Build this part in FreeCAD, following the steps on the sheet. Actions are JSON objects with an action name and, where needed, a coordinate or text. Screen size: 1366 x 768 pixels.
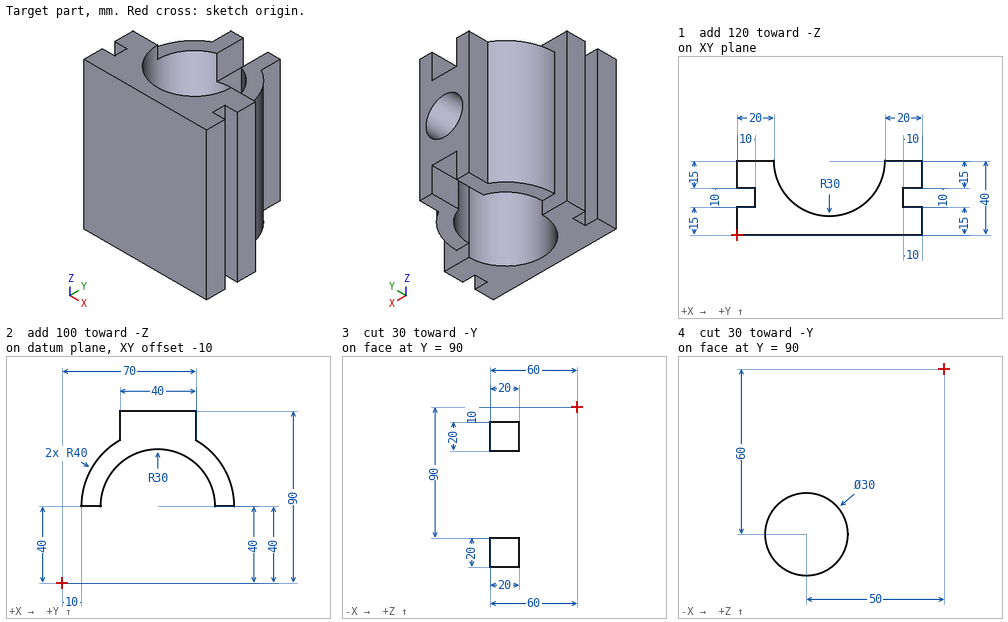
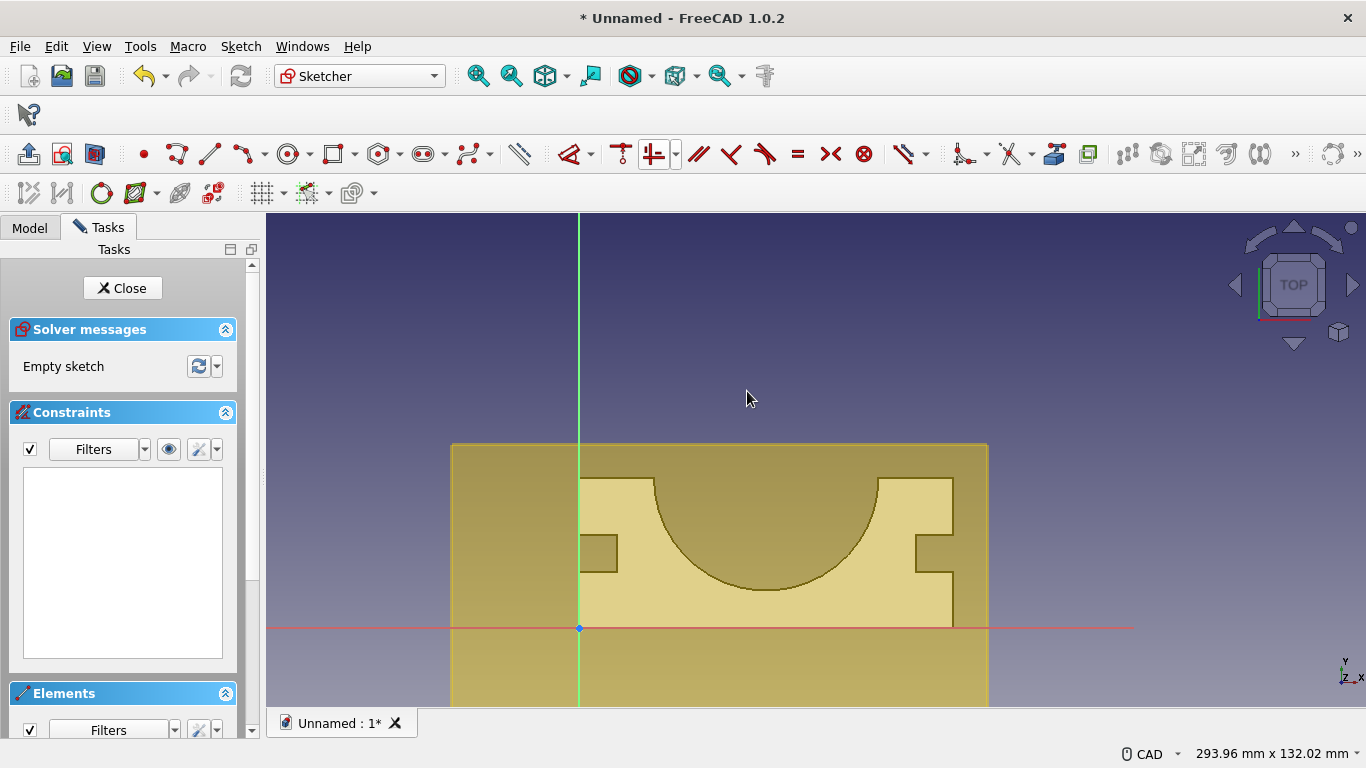
{"action": "left_click", "coordinate": [210, 154]}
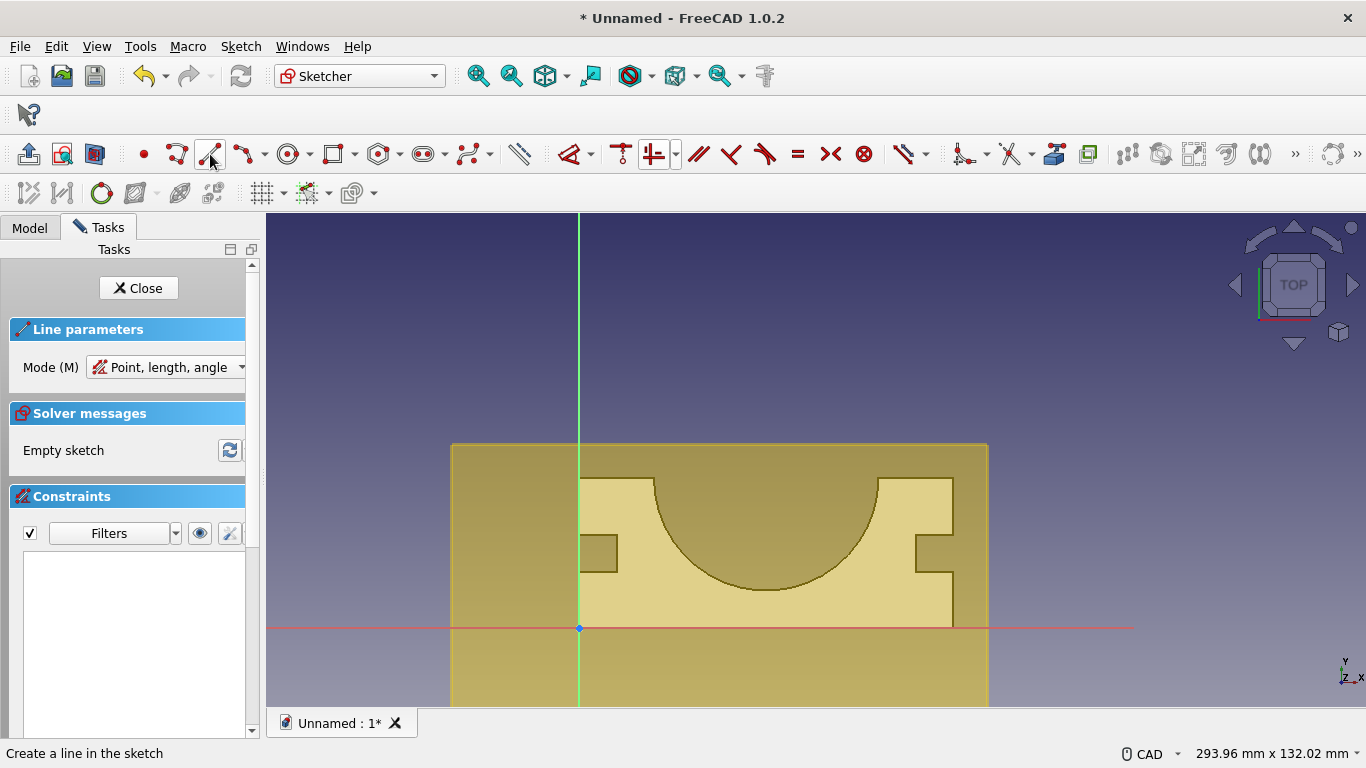
{"action": "left_click", "coordinate": [617, 478]}
{"action": "left_click", "coordinate": [654, 478]}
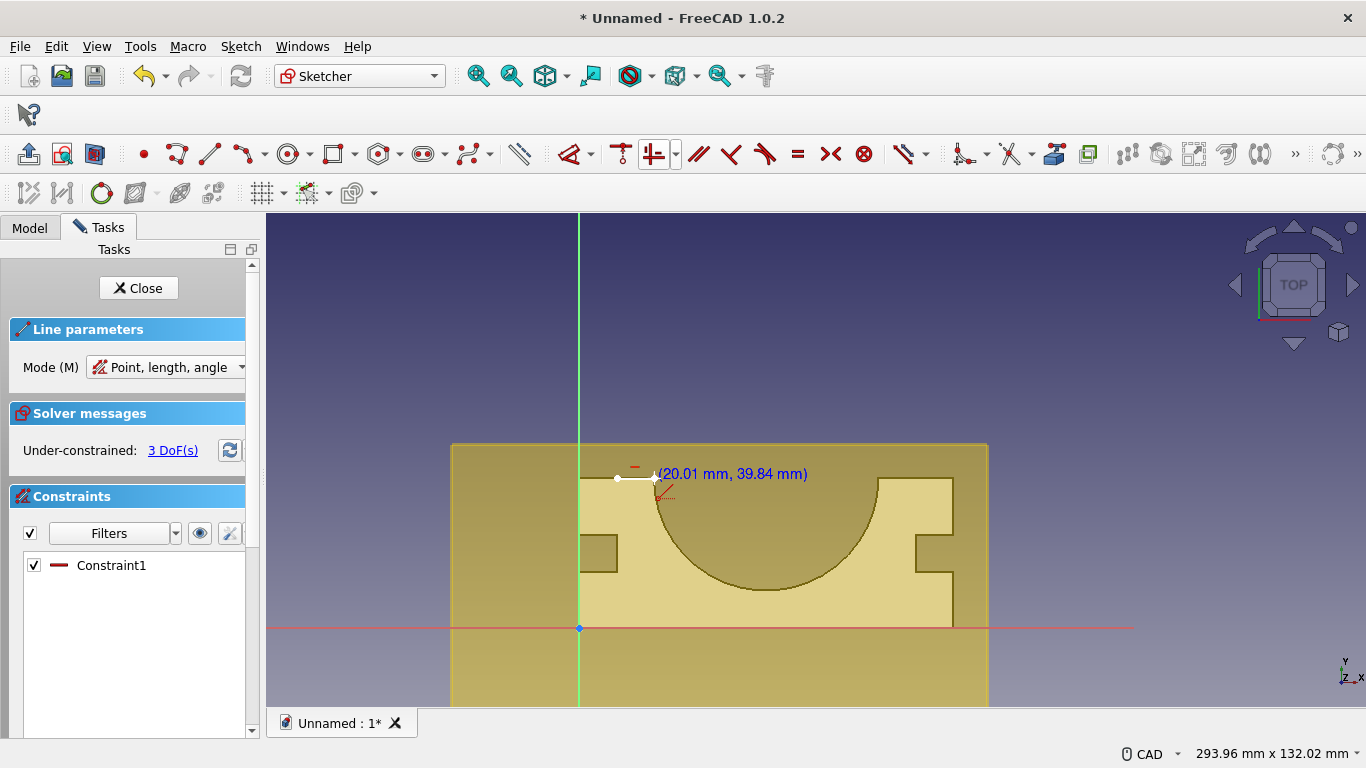
{"action": "left_click", "coordinate": [878, 478]}
{"action": "left_click", "coordinate": [916, 478]}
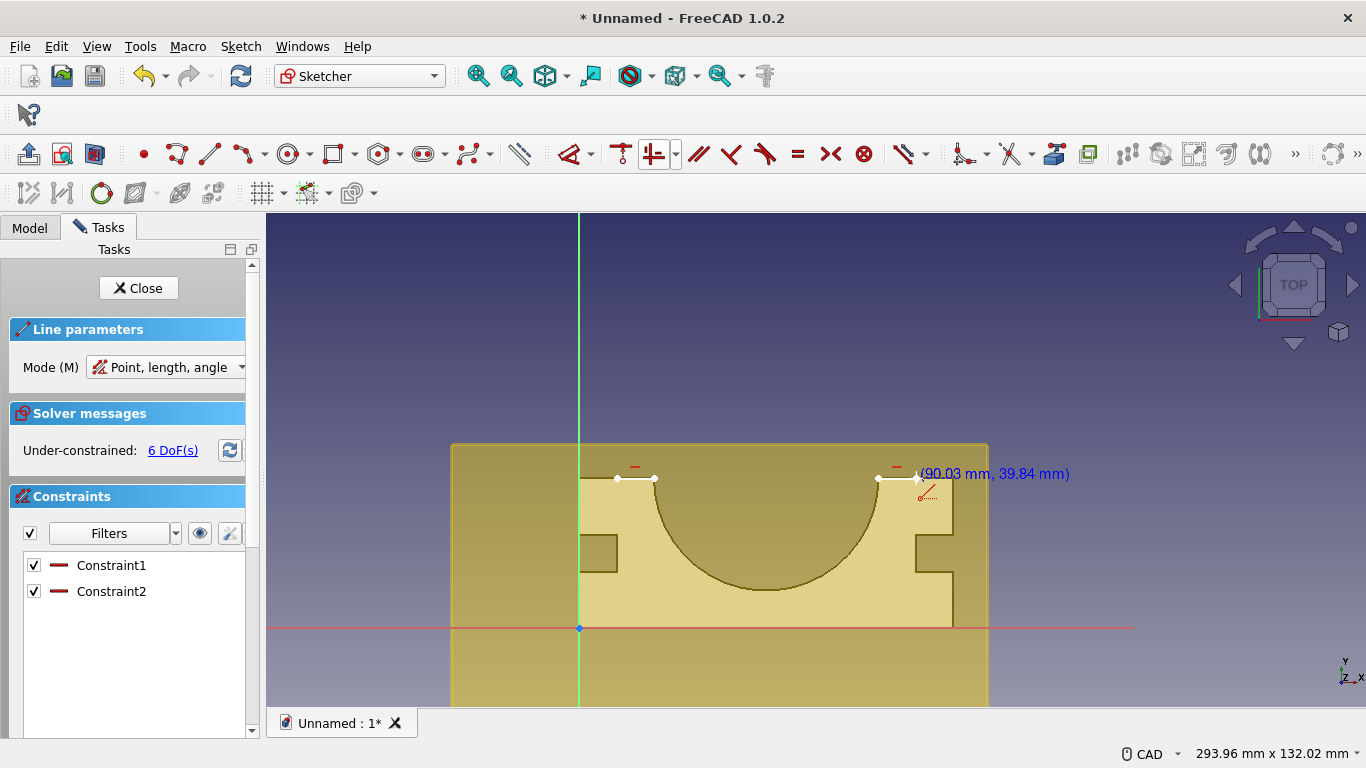
{"action": "left_click", "coordinate": [177, 154]}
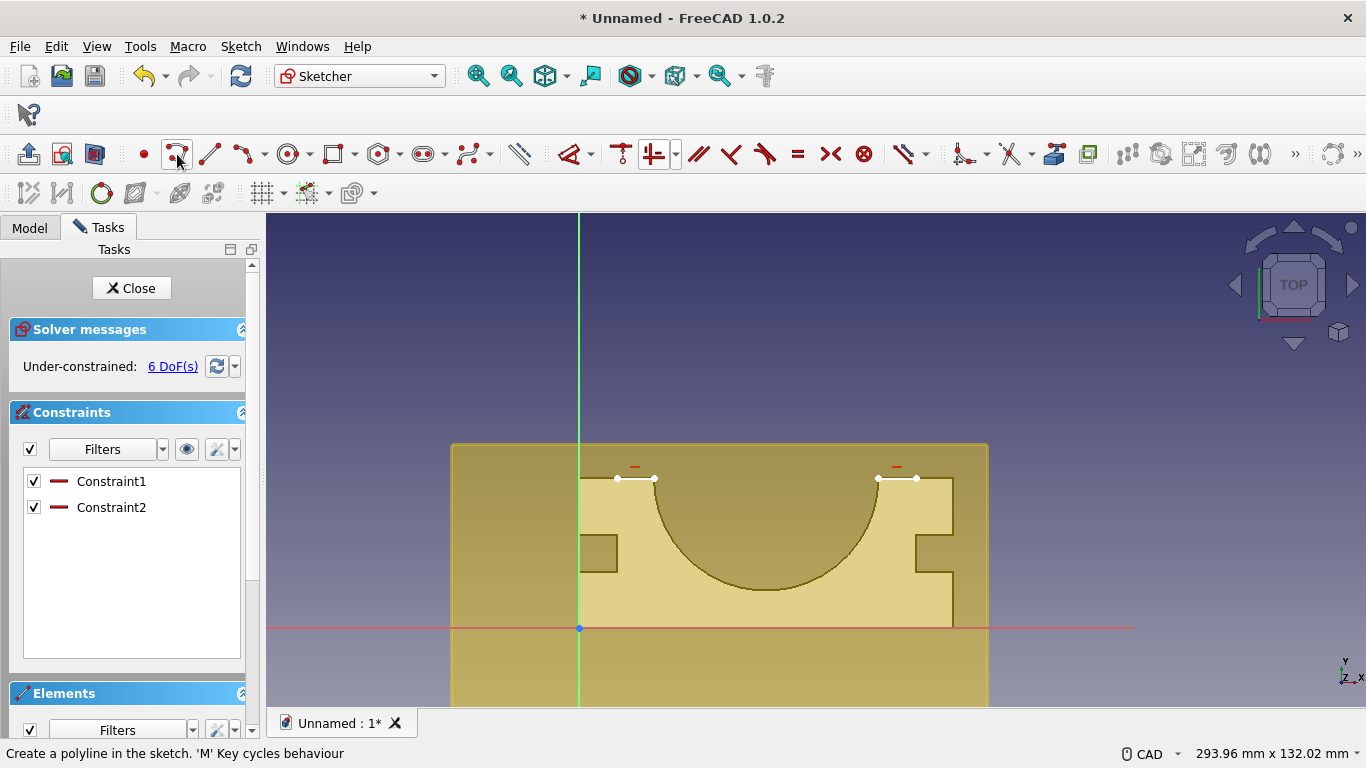
{"action": "left_click", "coordinate": [841, 349]}
{"action": "left_click", "coordinate": [841, 291]}
{"action": "left_click", "coordinate": [691, 291]}
{"action": "left_click", "coordinate": [691, 349]}
{"action": "right_click", "coordinate": [691, 349]}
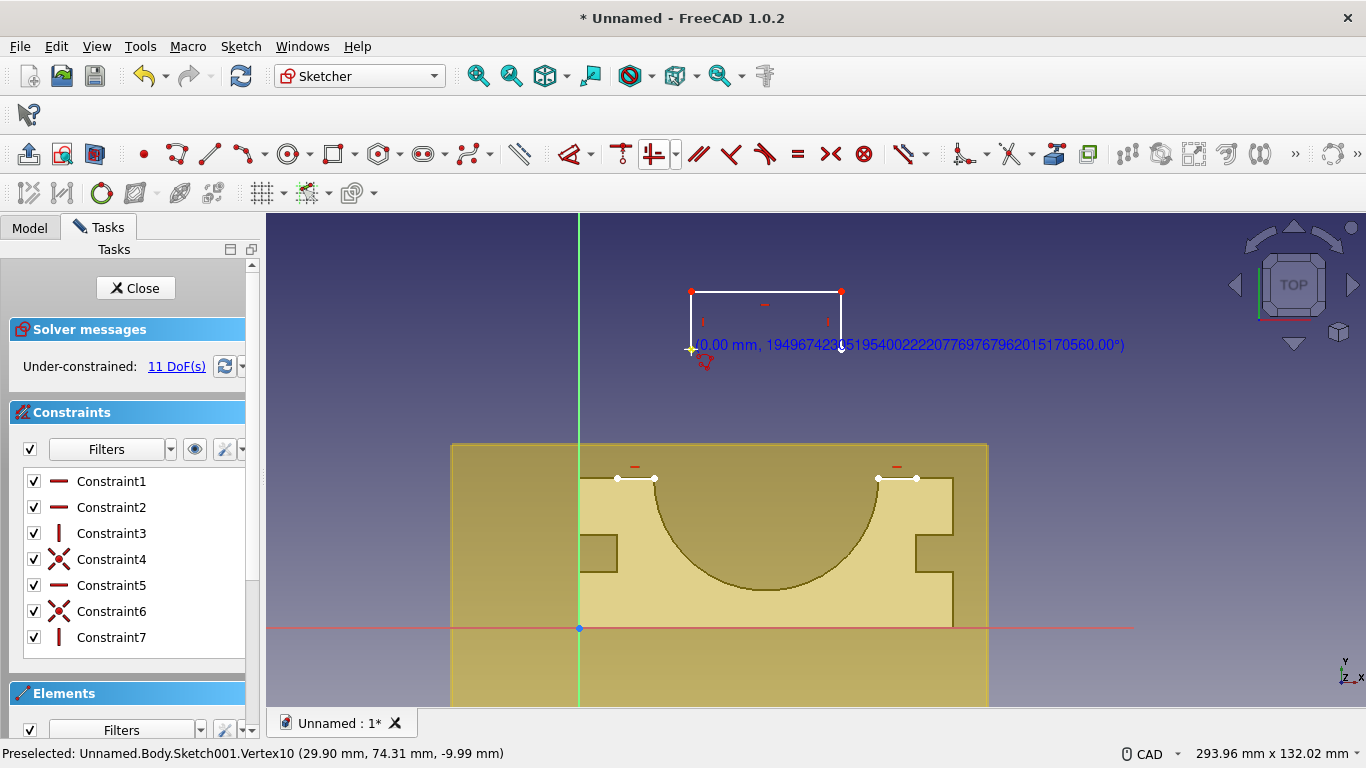
{"action": "left_click", "coordinate": [242, 154]}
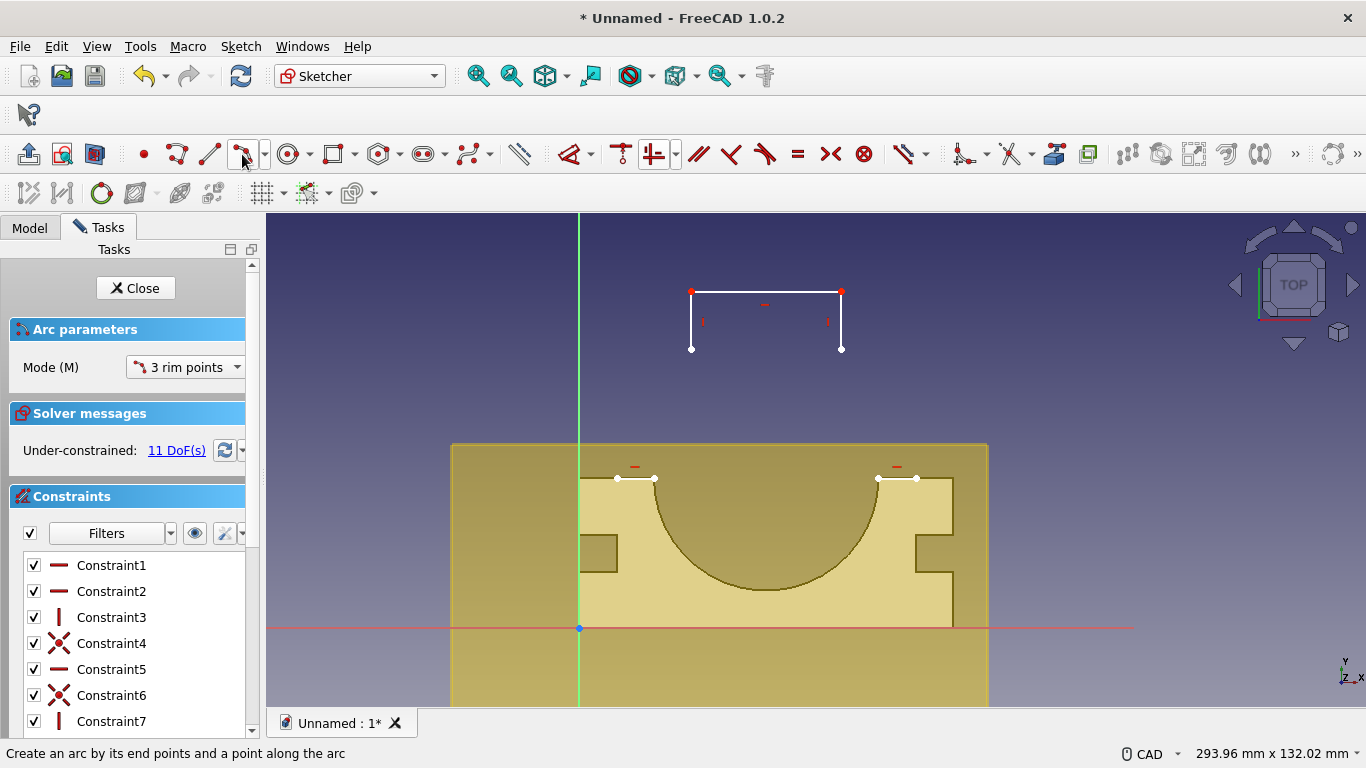
{"action": "left_click", "coordinate": [654, 479]}
{"action": "left_click", "coordinate": [878, 479]}
{"action": "left_click", "coordinate": [766, 366]}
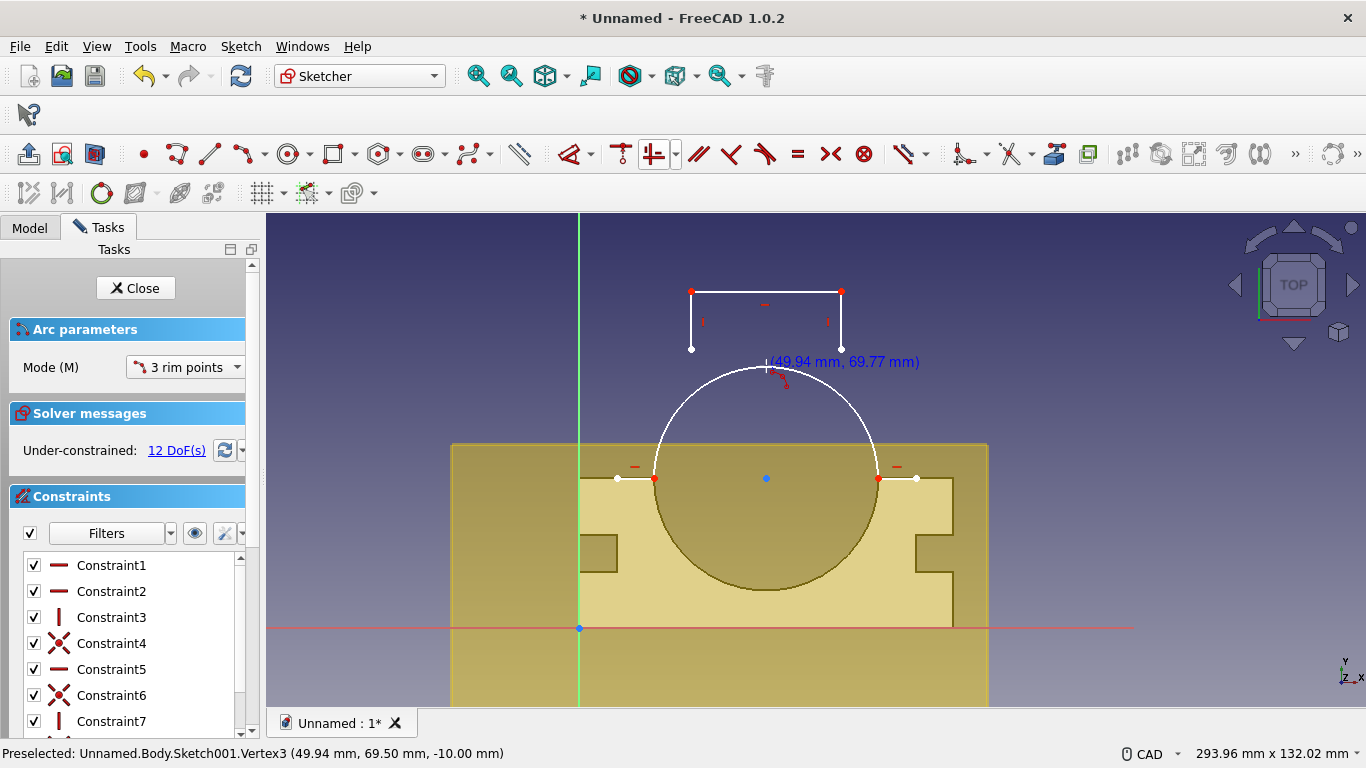
{"action": "left_click", "coordinate": [916, 479]}
{"action": "left_click", "coordinate": [841, 350]}
{"action": "left_click", "coordinate": [896, 404]}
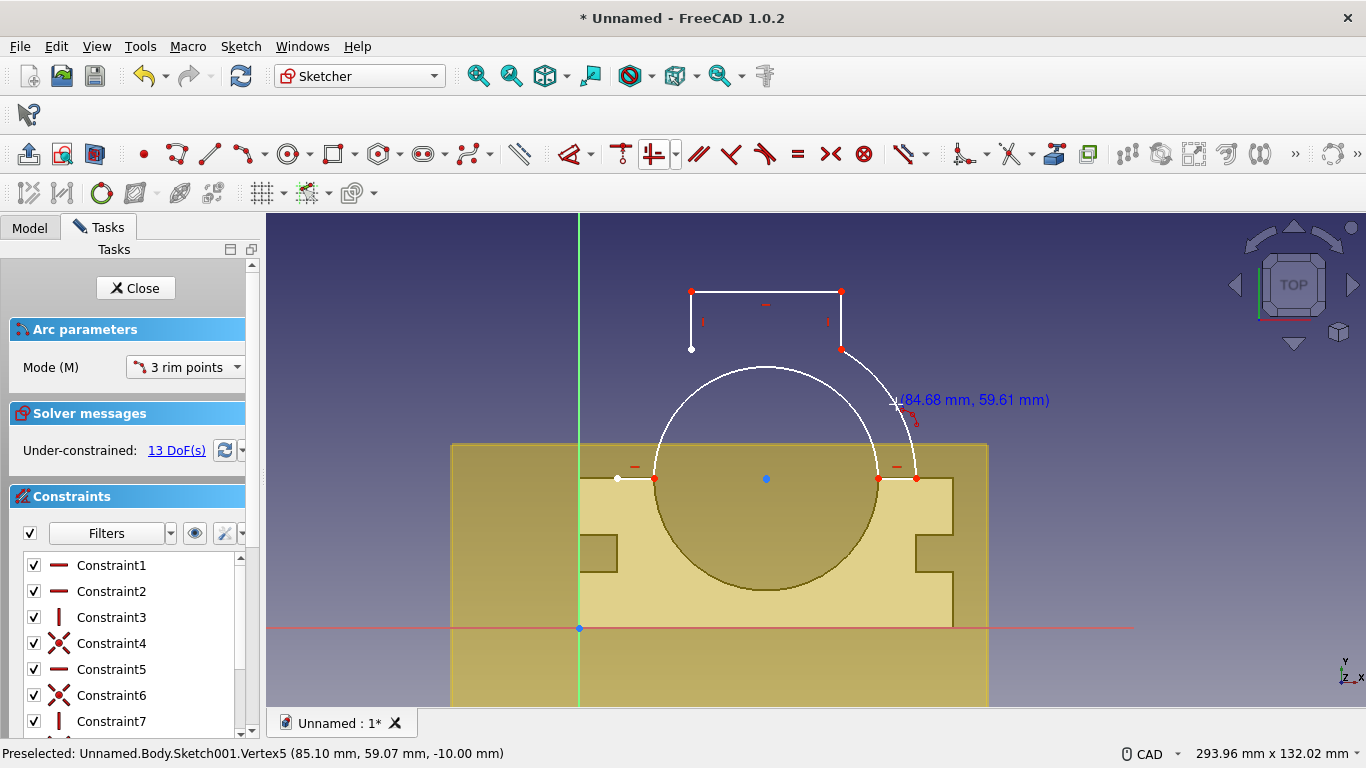
{"action": "left_click", "coordinate": [691, 350]}
{"action": "left_click", "coordinate": [617, 479]}
{"action": "left_click", "coordinate": [637, 404]}
{"action": "key", "text": "Escape"}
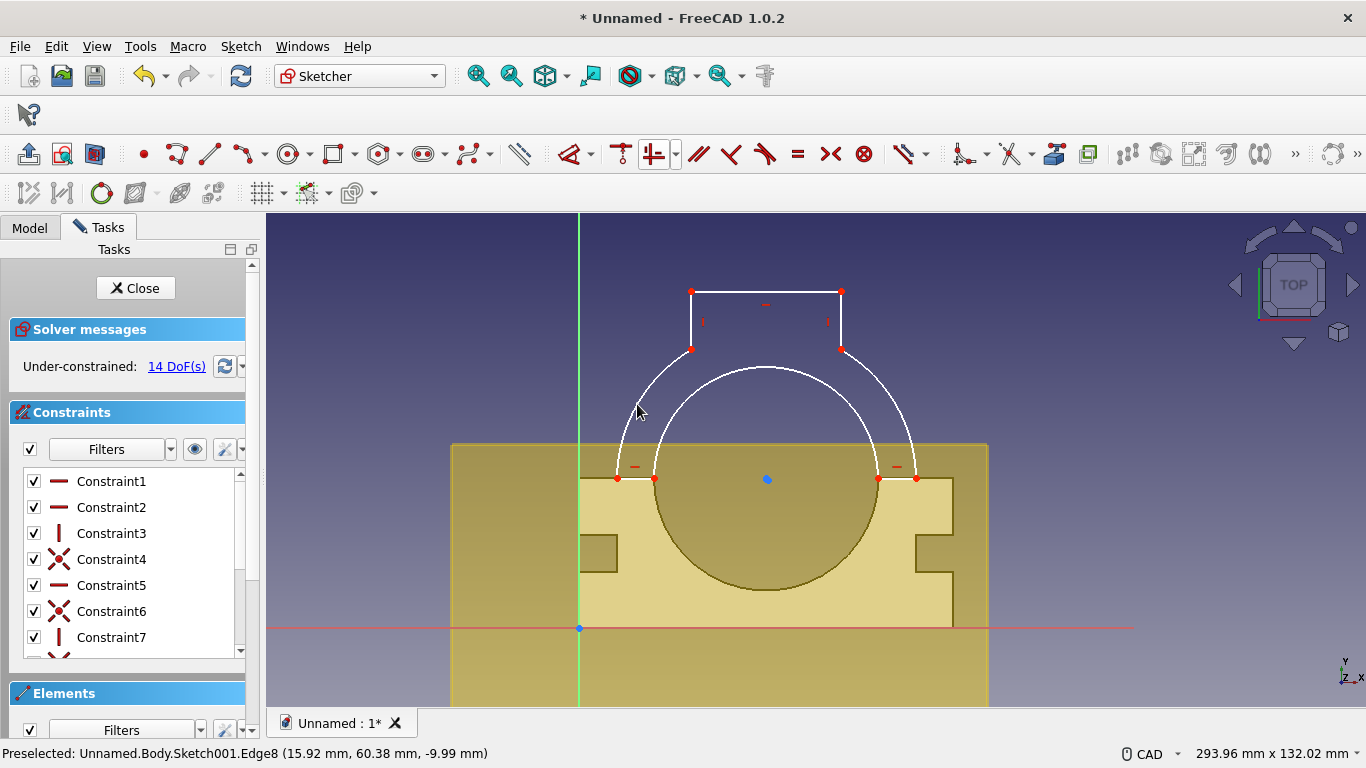
{"action": "left_click", "coordinate": [832, 388]}